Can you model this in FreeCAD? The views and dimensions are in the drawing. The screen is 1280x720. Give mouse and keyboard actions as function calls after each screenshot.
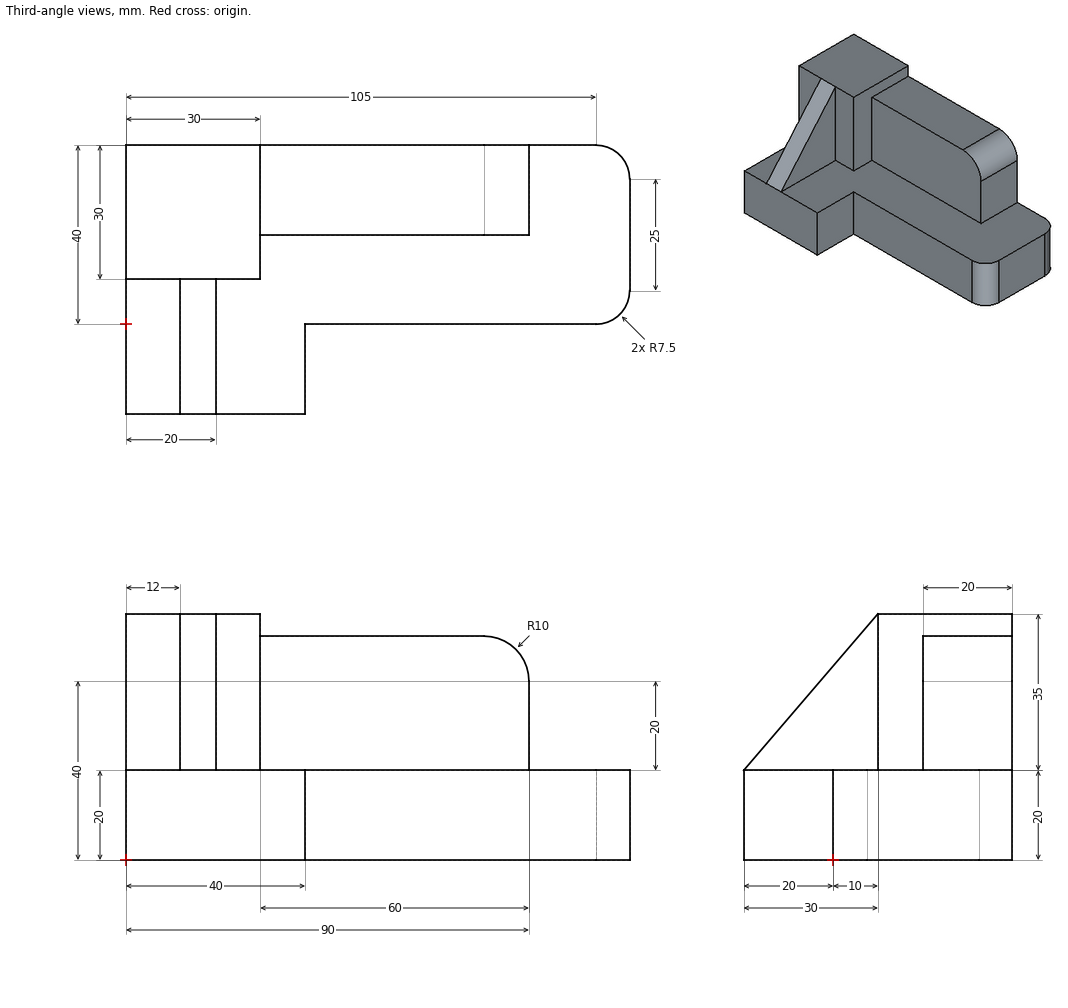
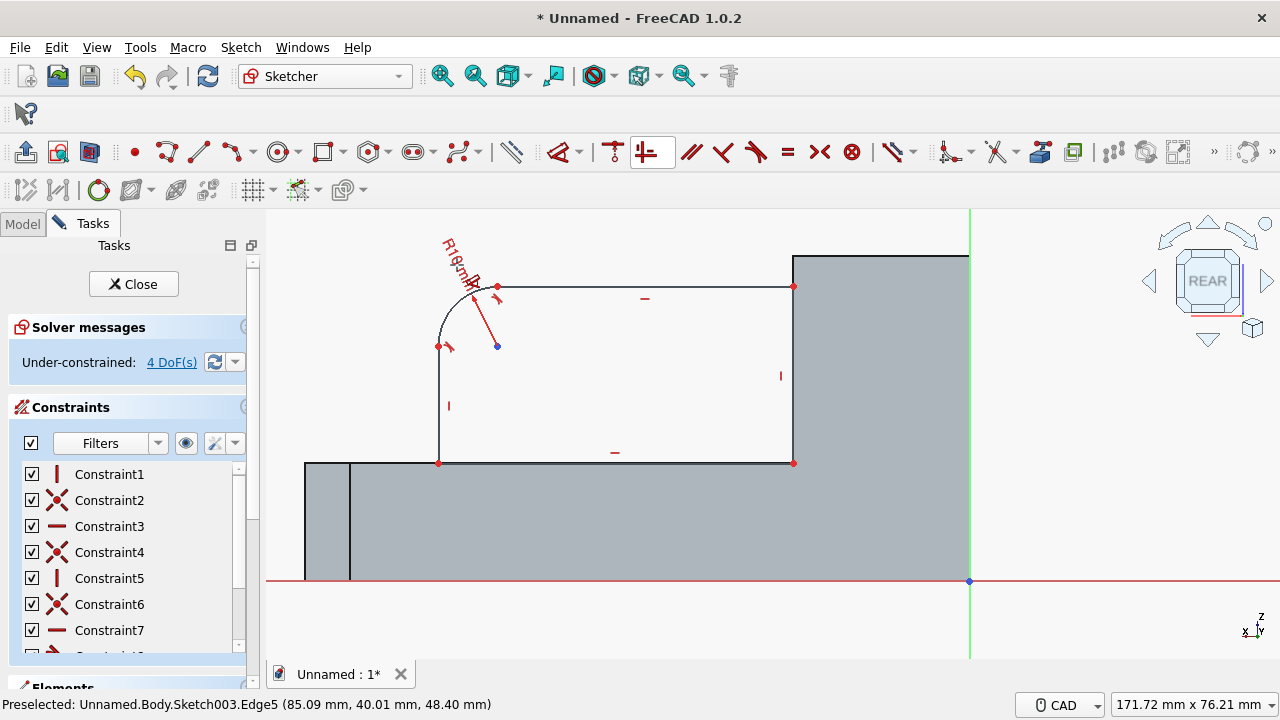
click(439, 381)
click(405, 405)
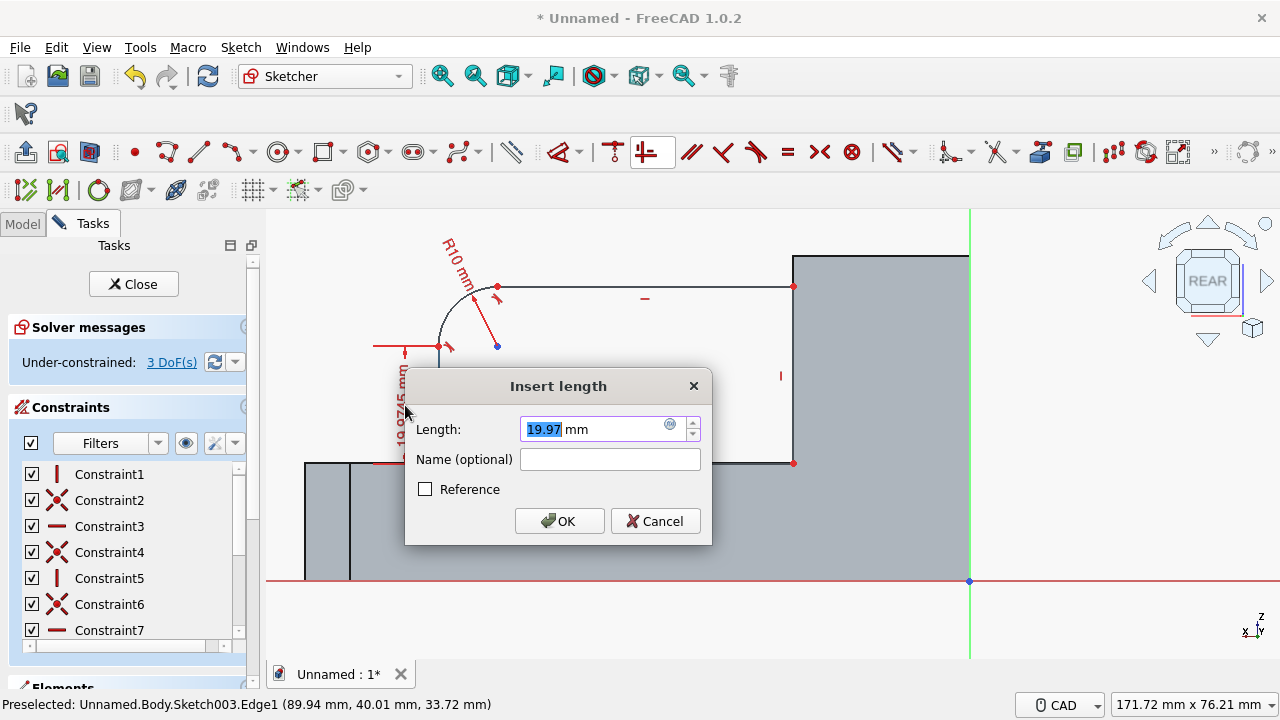
text(20)
key(Return)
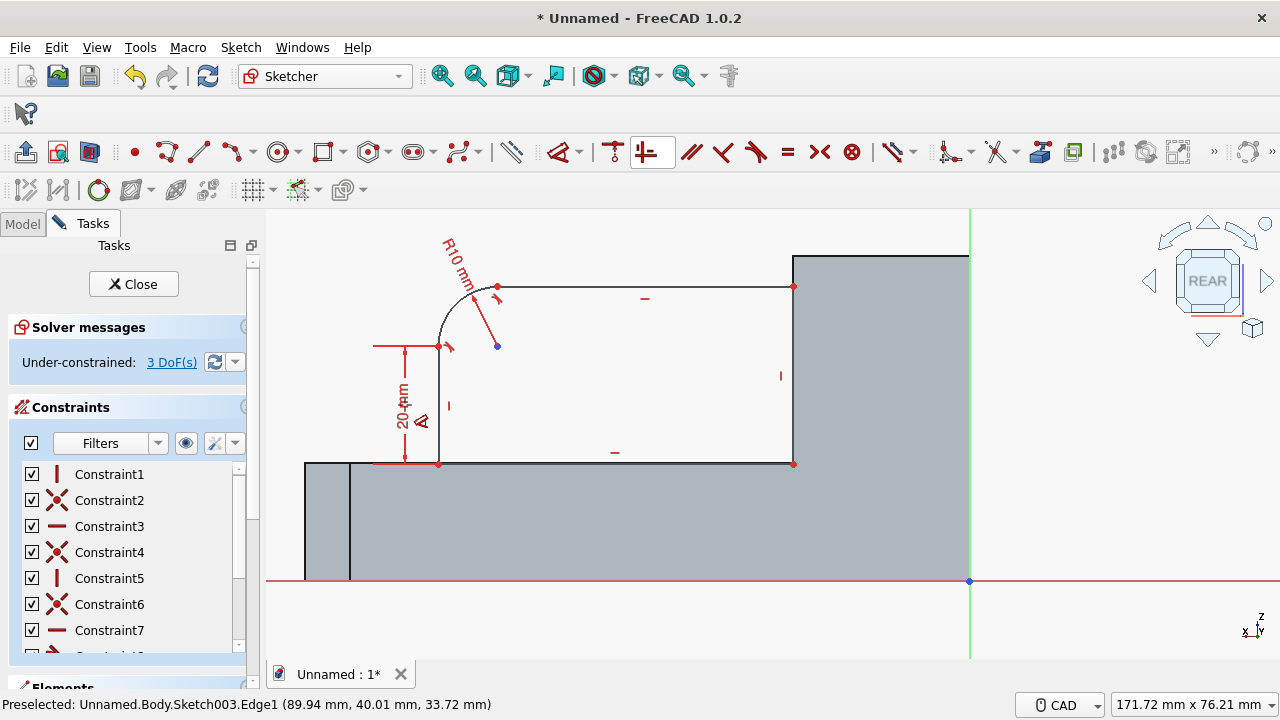
click(545, 464)
click(616, 498)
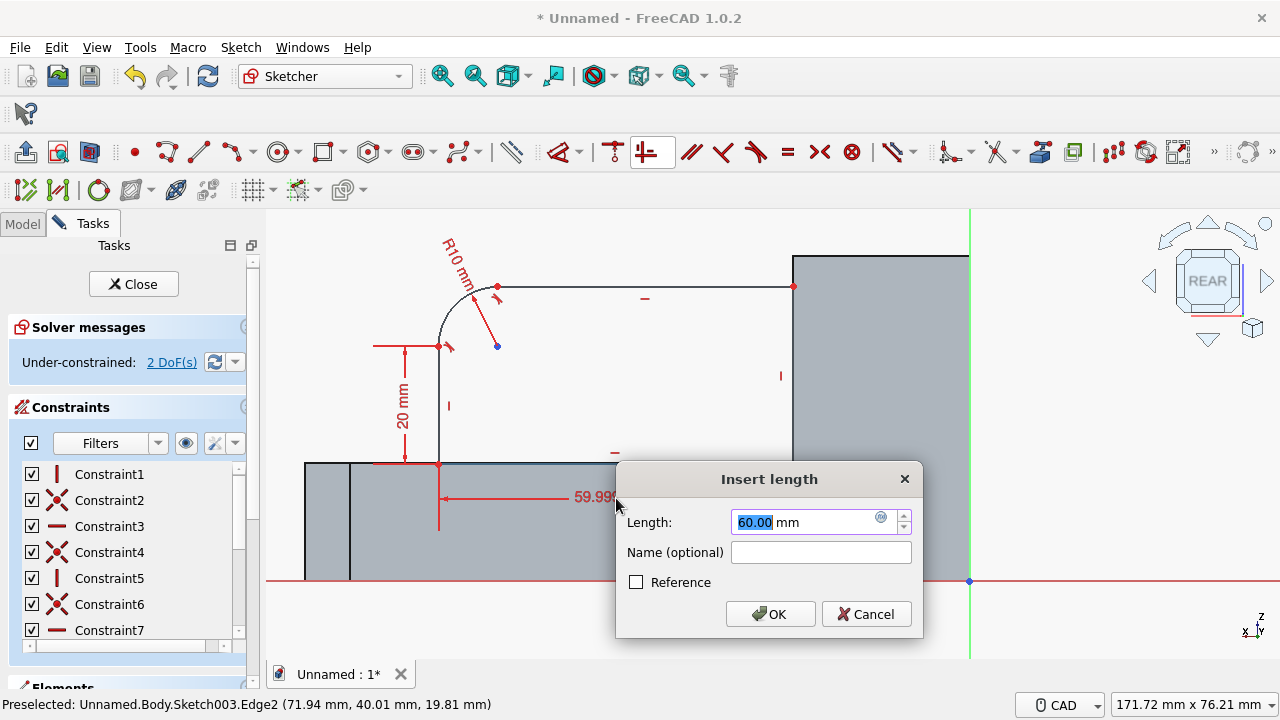
text(60)
key(Return)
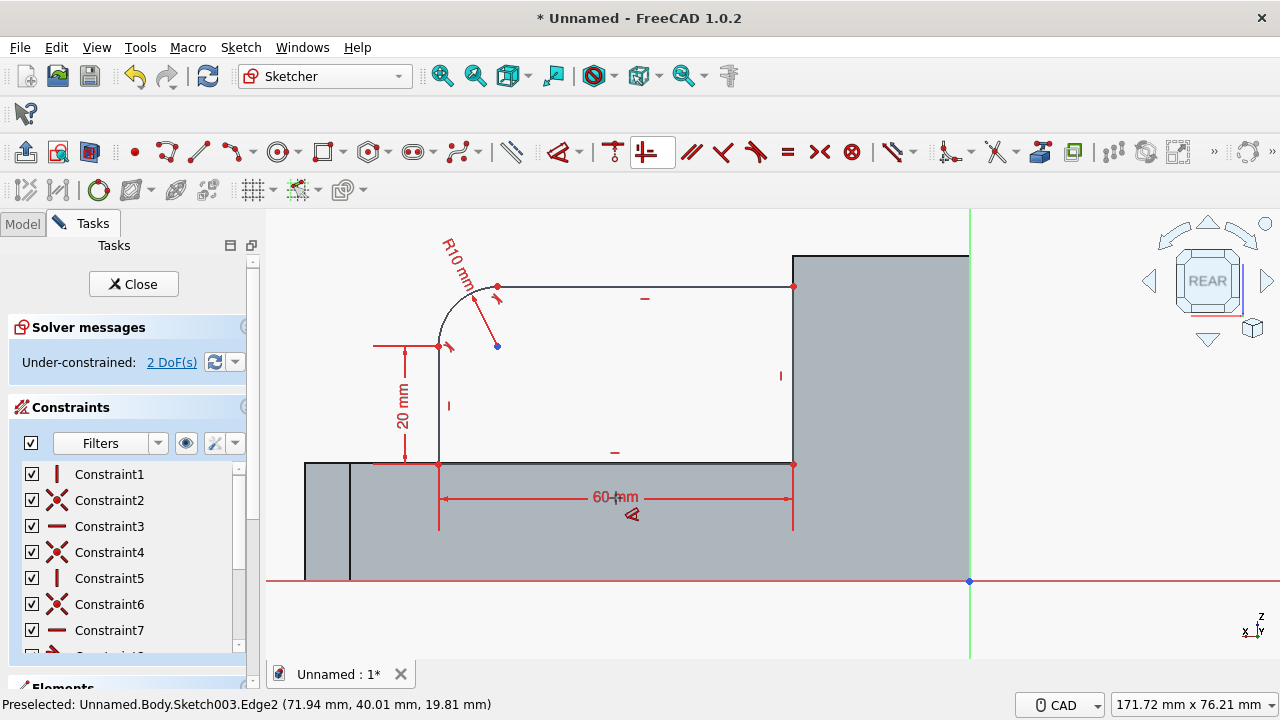
click(439, 346)
click(704, 615)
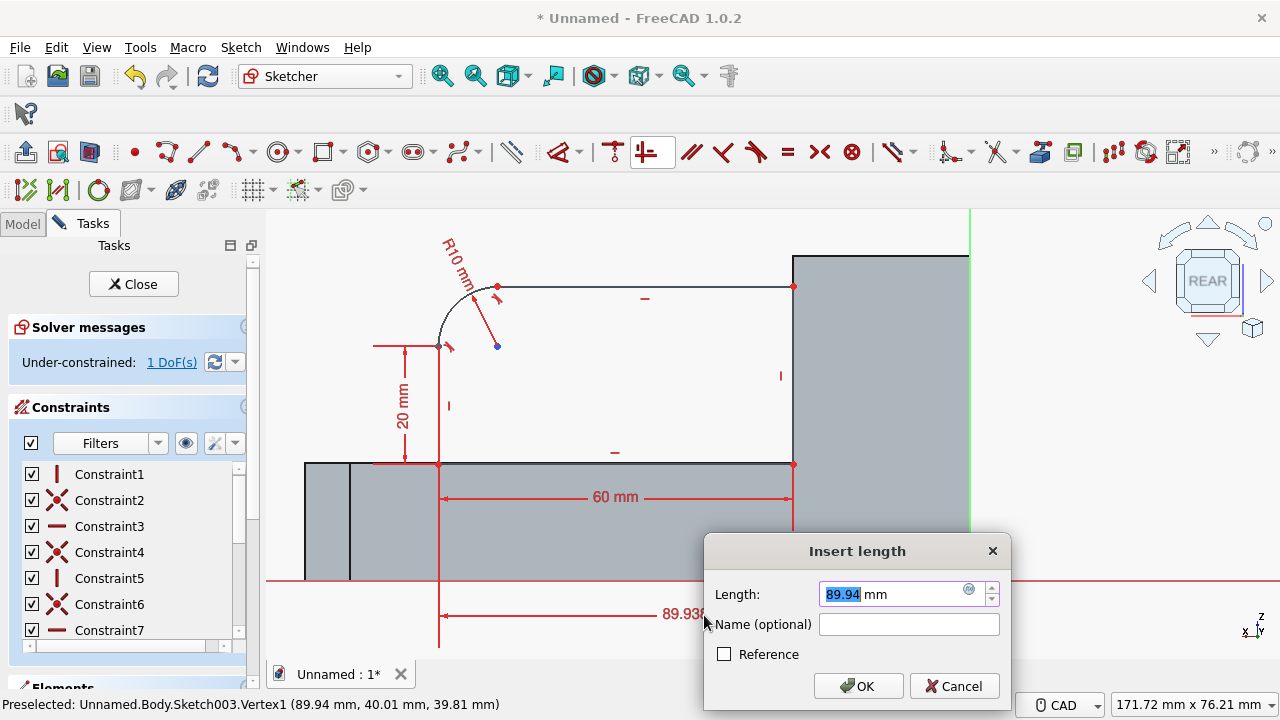
text(90)
key(Return)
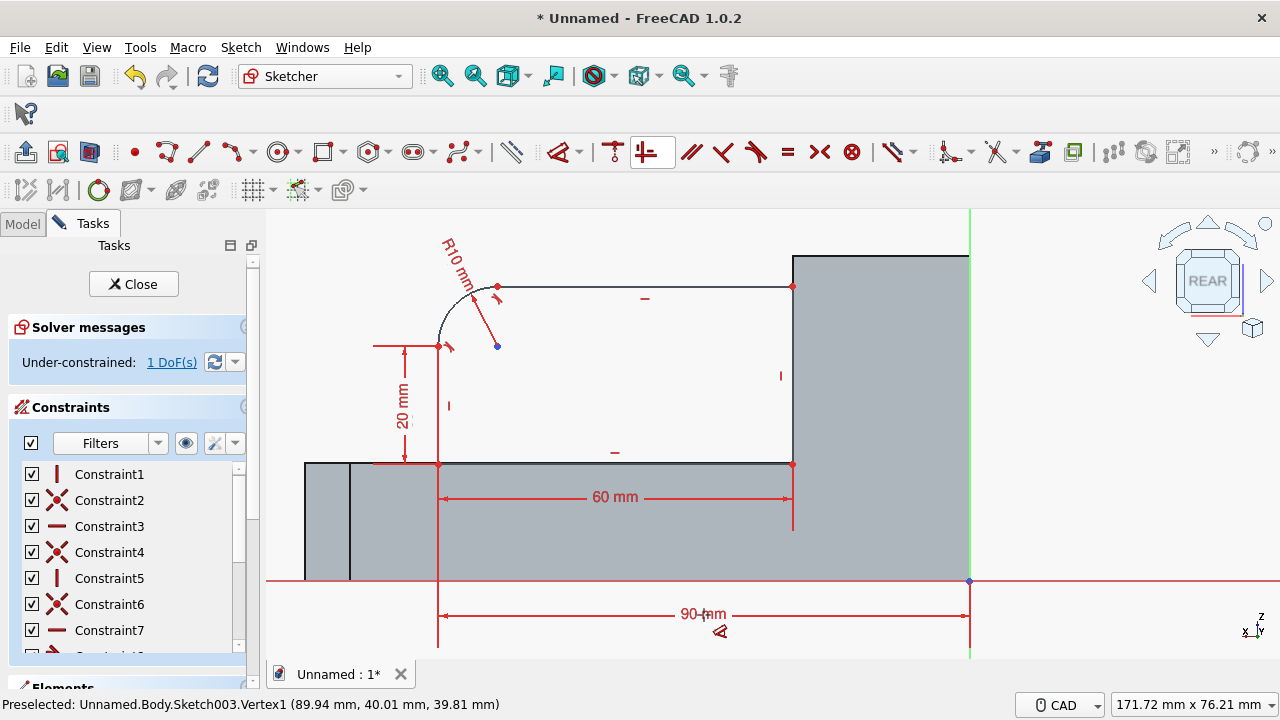
click(438, 346)
click(1004, 464)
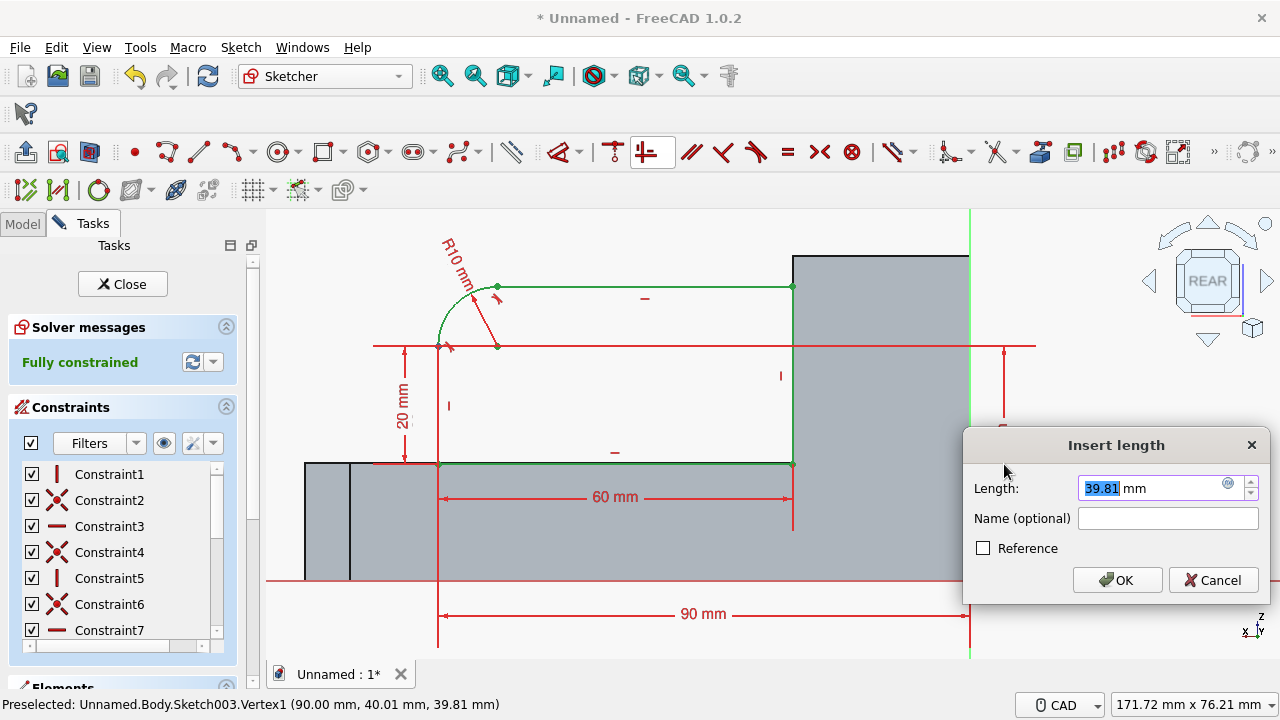
text(40)
key(Return)
key(Escape)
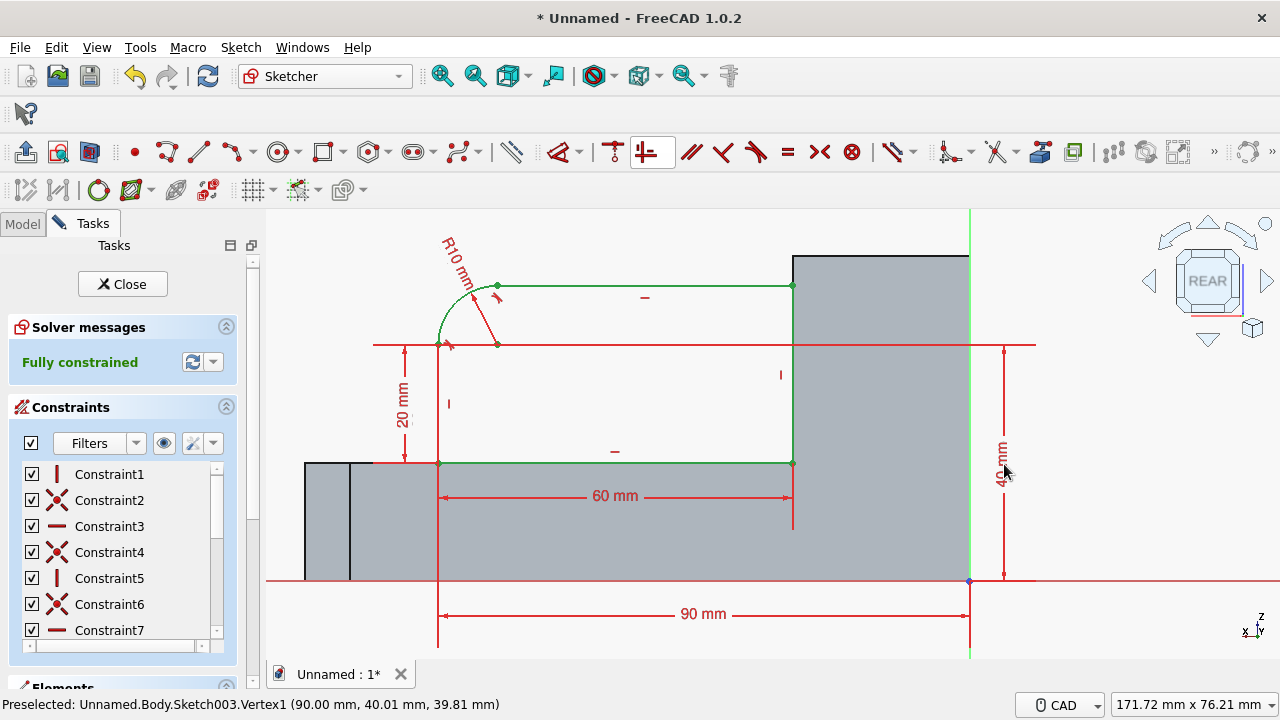
click(123, 284)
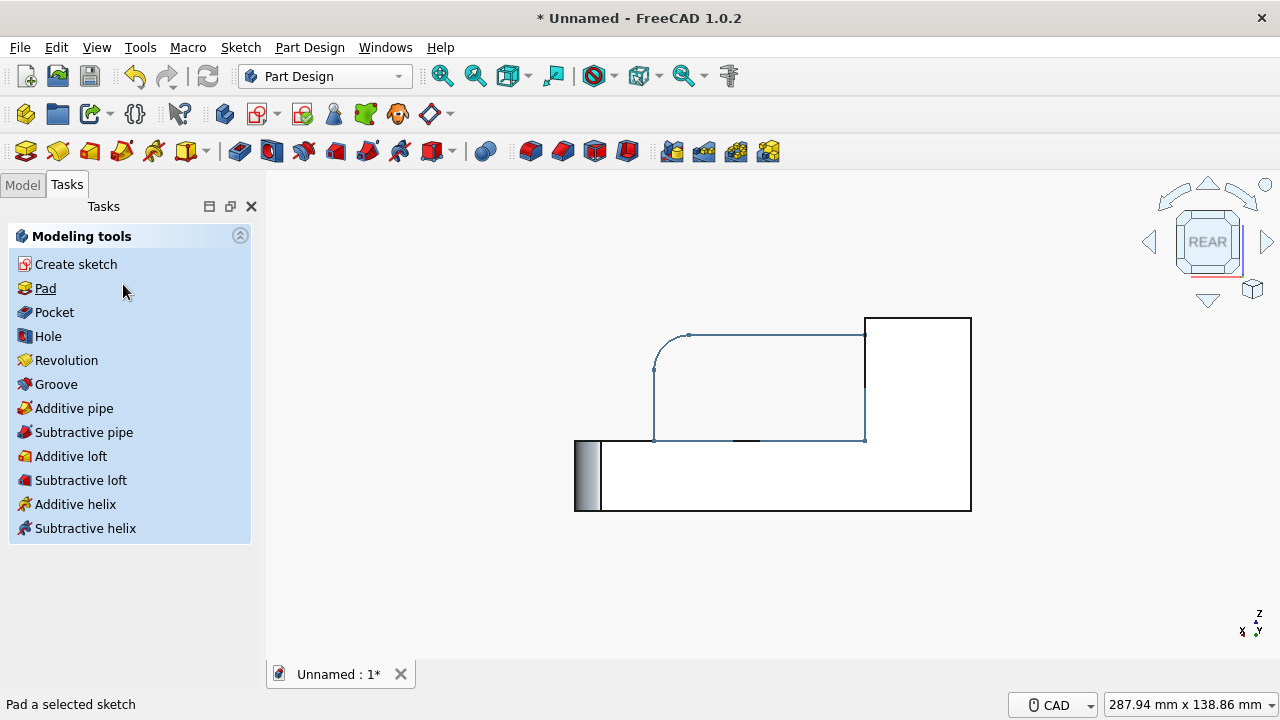
click(26, 152)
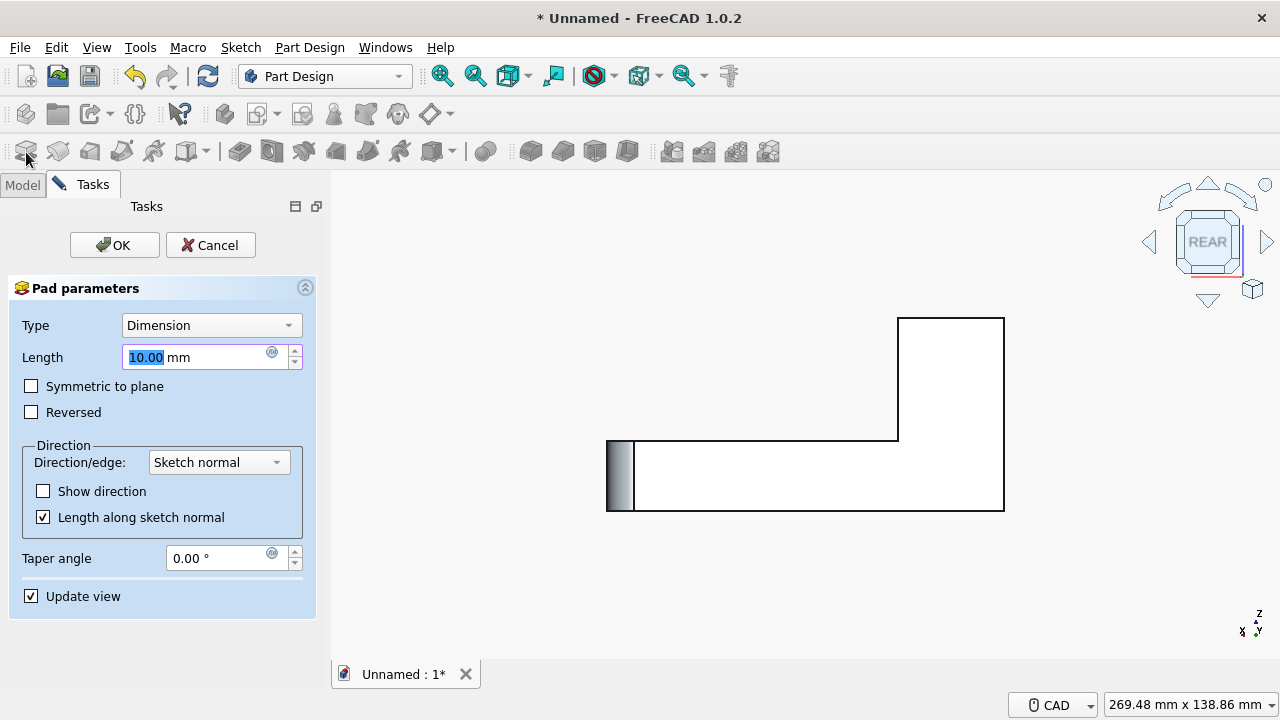
text(20)
key(Tab)